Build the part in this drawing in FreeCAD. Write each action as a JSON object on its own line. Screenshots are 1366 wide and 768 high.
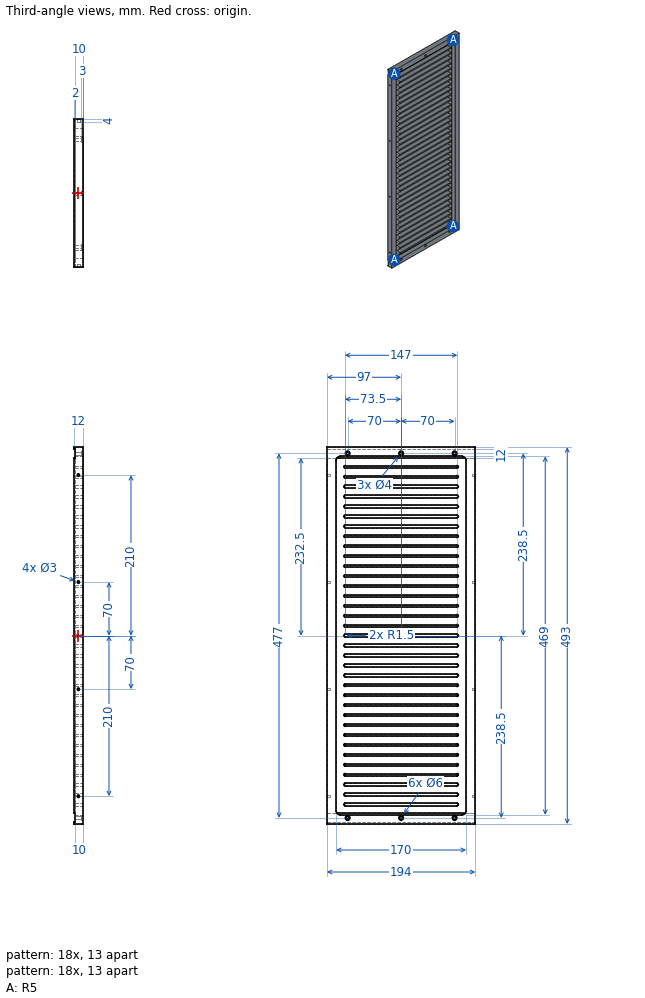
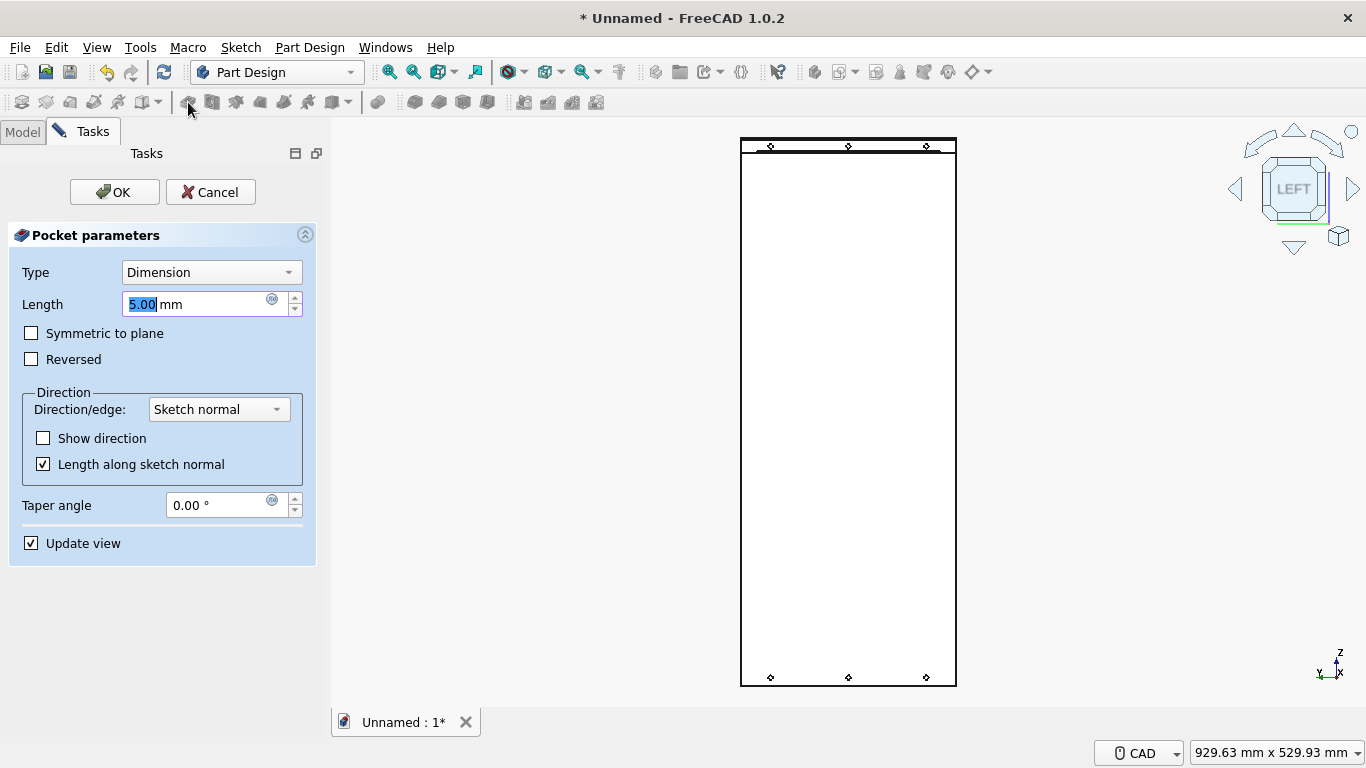
{"action": "type", "text": "2"}
{"action": "key", "text": "Tab"}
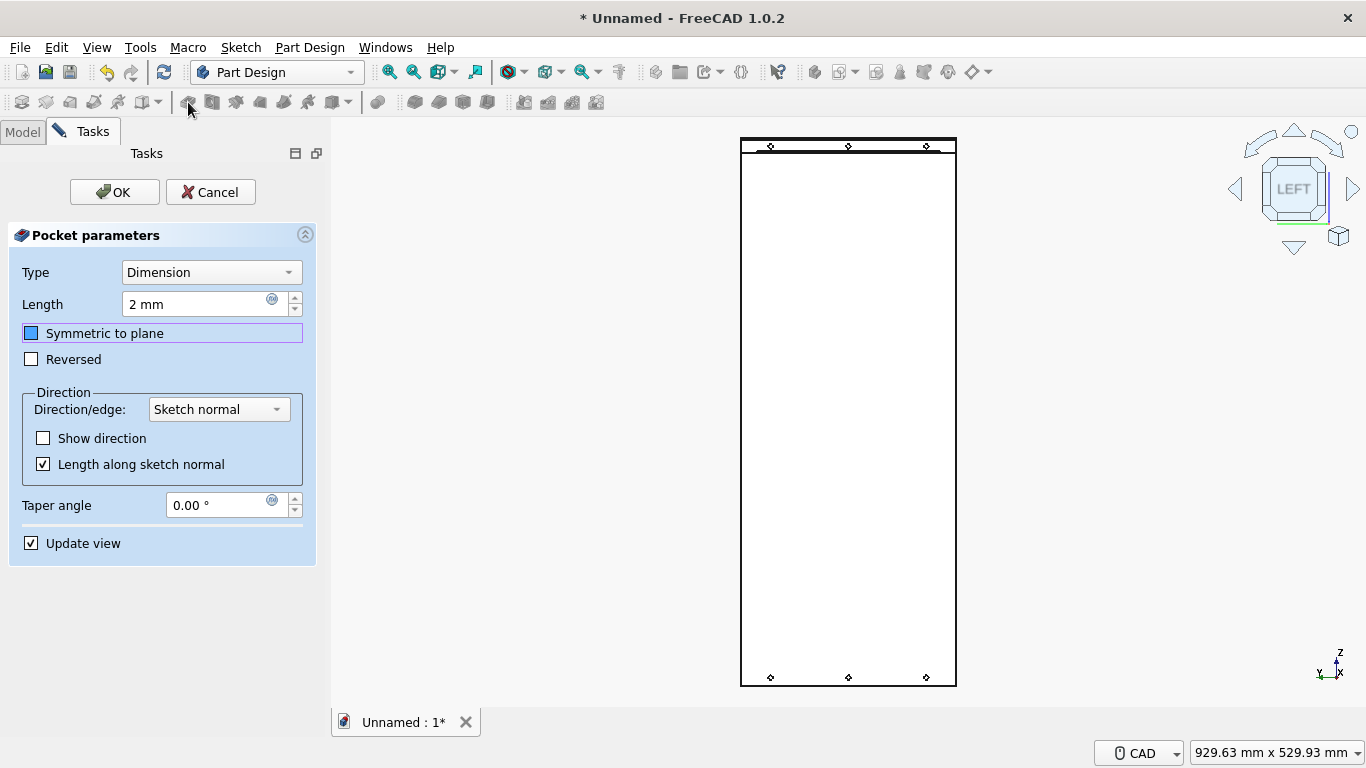
{"action": "left_click", "coordinate": [115, 192]}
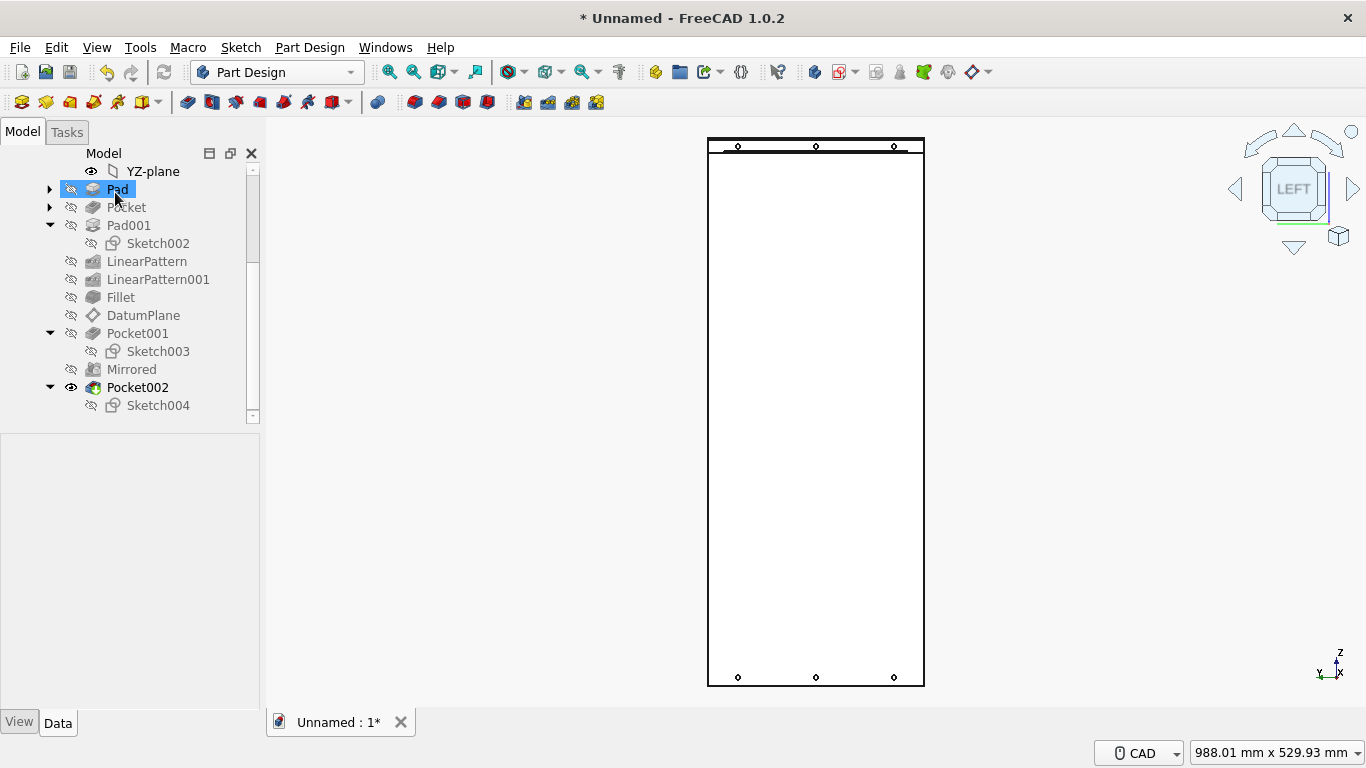
{"action": "left_click", "coordinate": [116, 387]}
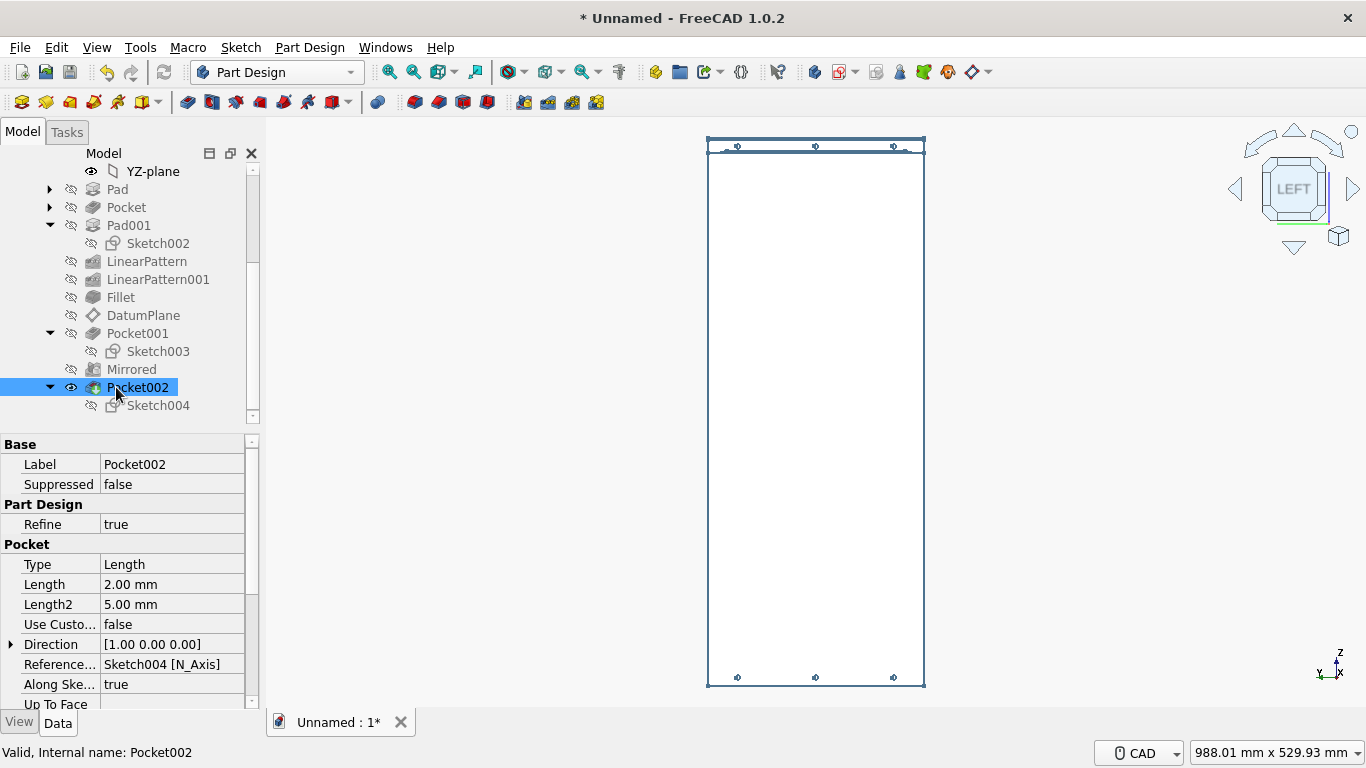
{"action": "left_click", "coordinate": [524, 102]}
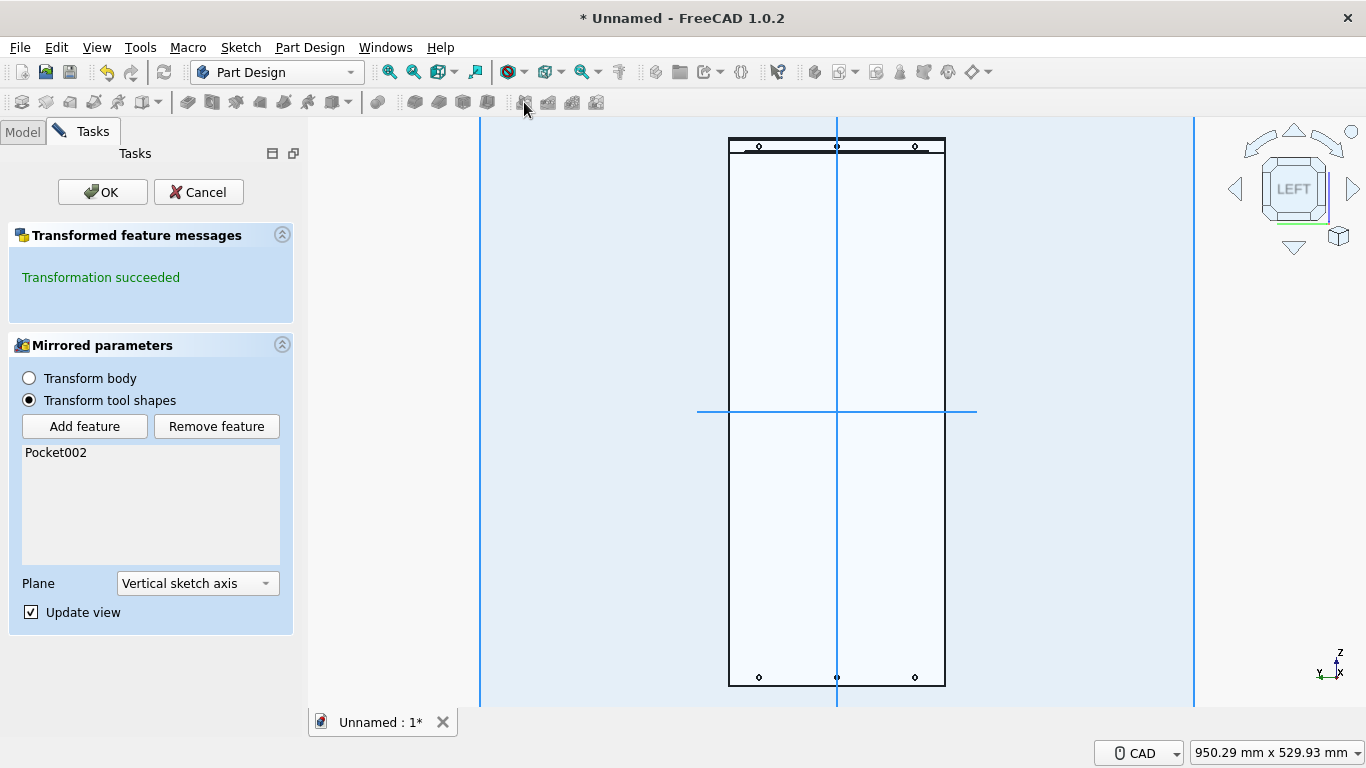
{"action": "left_click", "coordinate": [198, 584]}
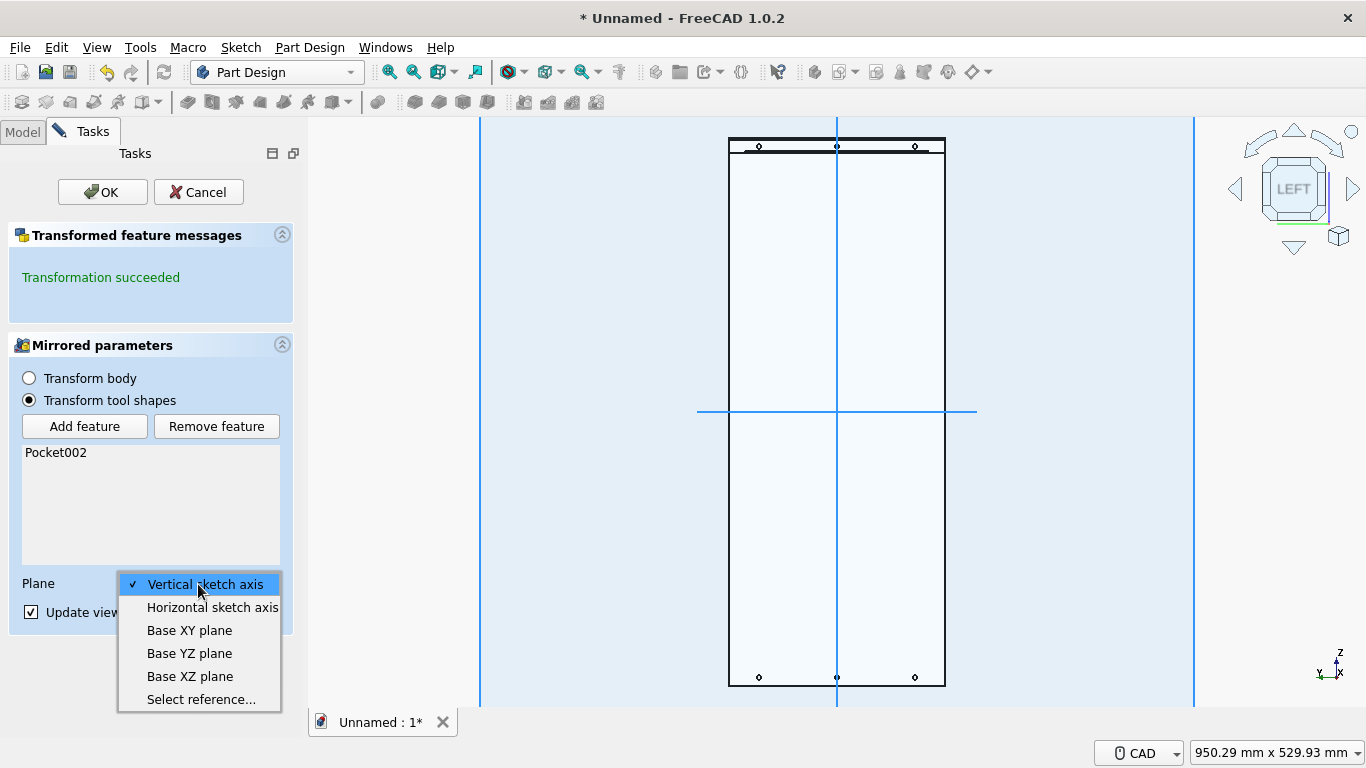
{"action": "left_click", "coordinate": [198, 630]}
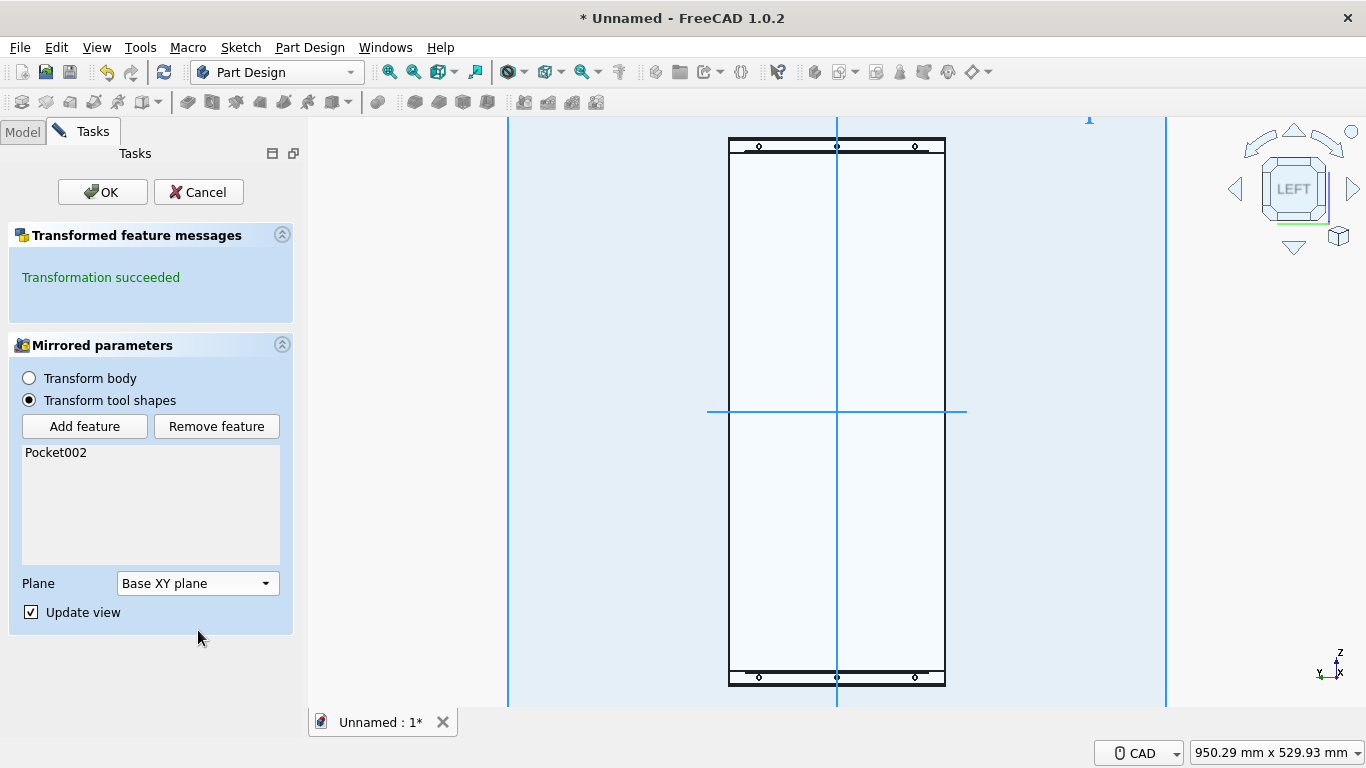
{"action": "left_click", "coordinate": [103, 192]}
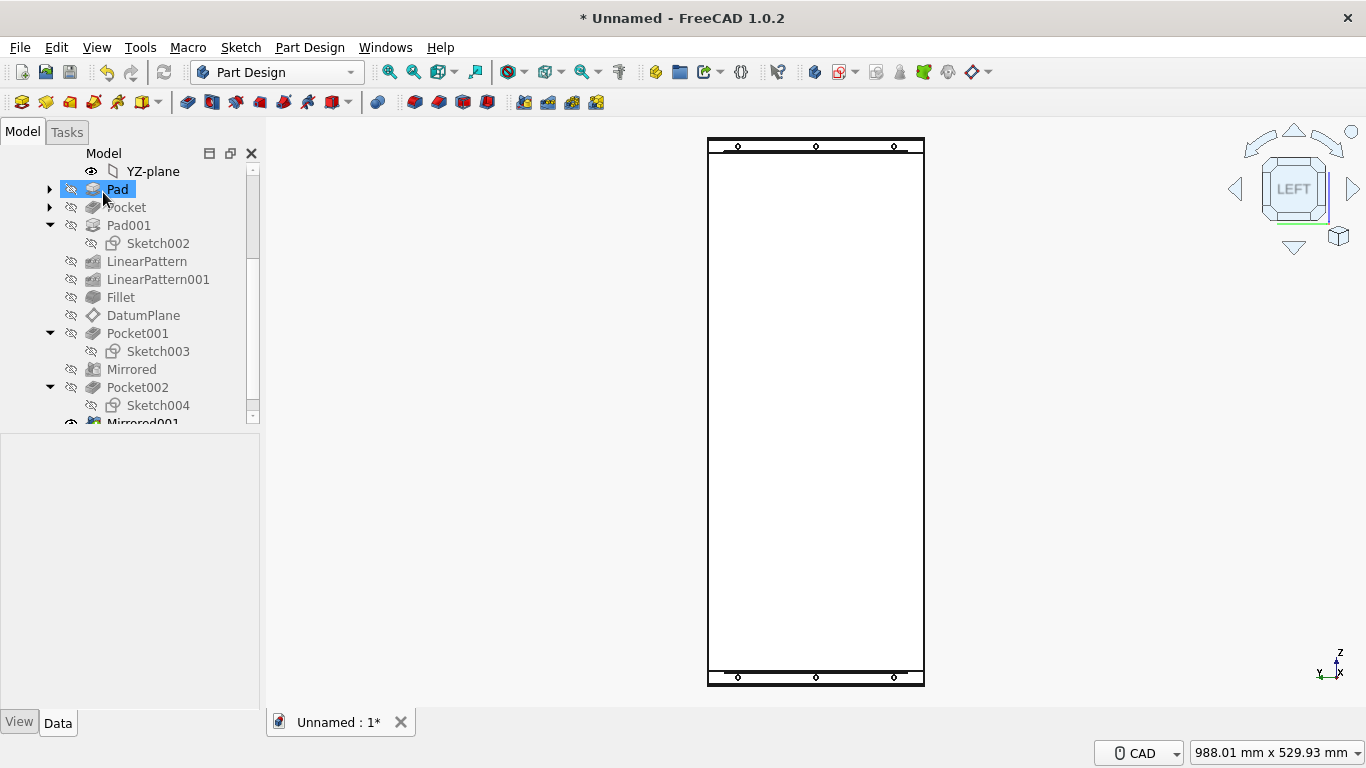
{"action": "key", "text": "4"}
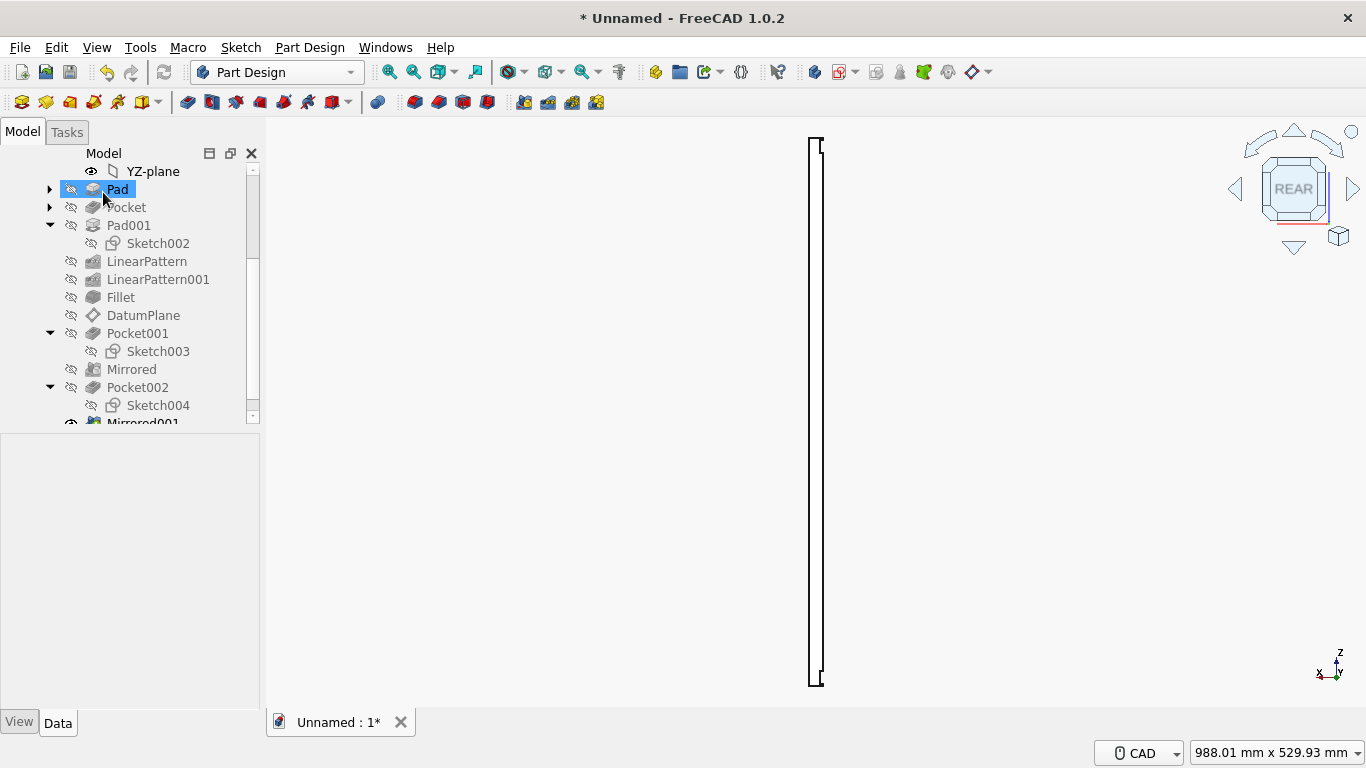
{"action": "scroll", "coordinate": [816, 568], "scroll_direction": "up", "scroll_amount": 3}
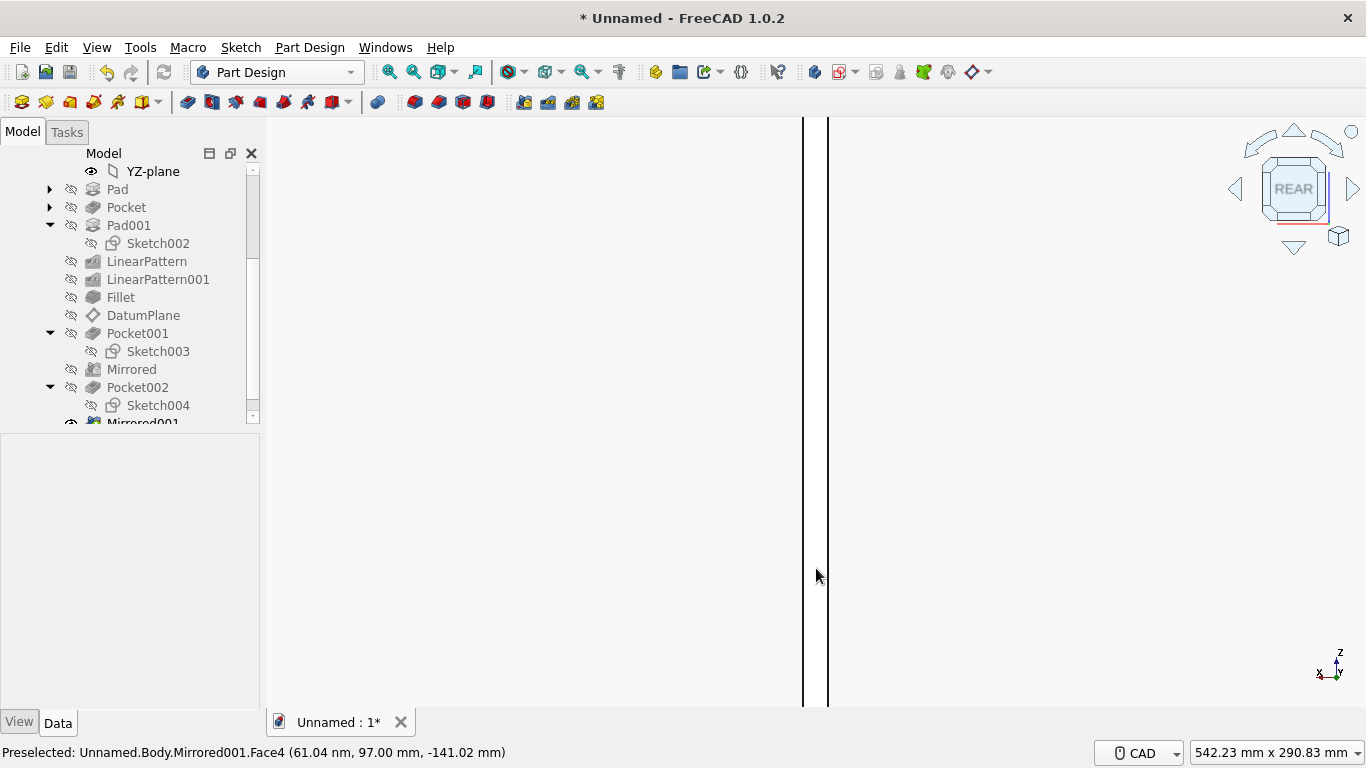
{"action": "left_click", "coordinate": [816, 568]}